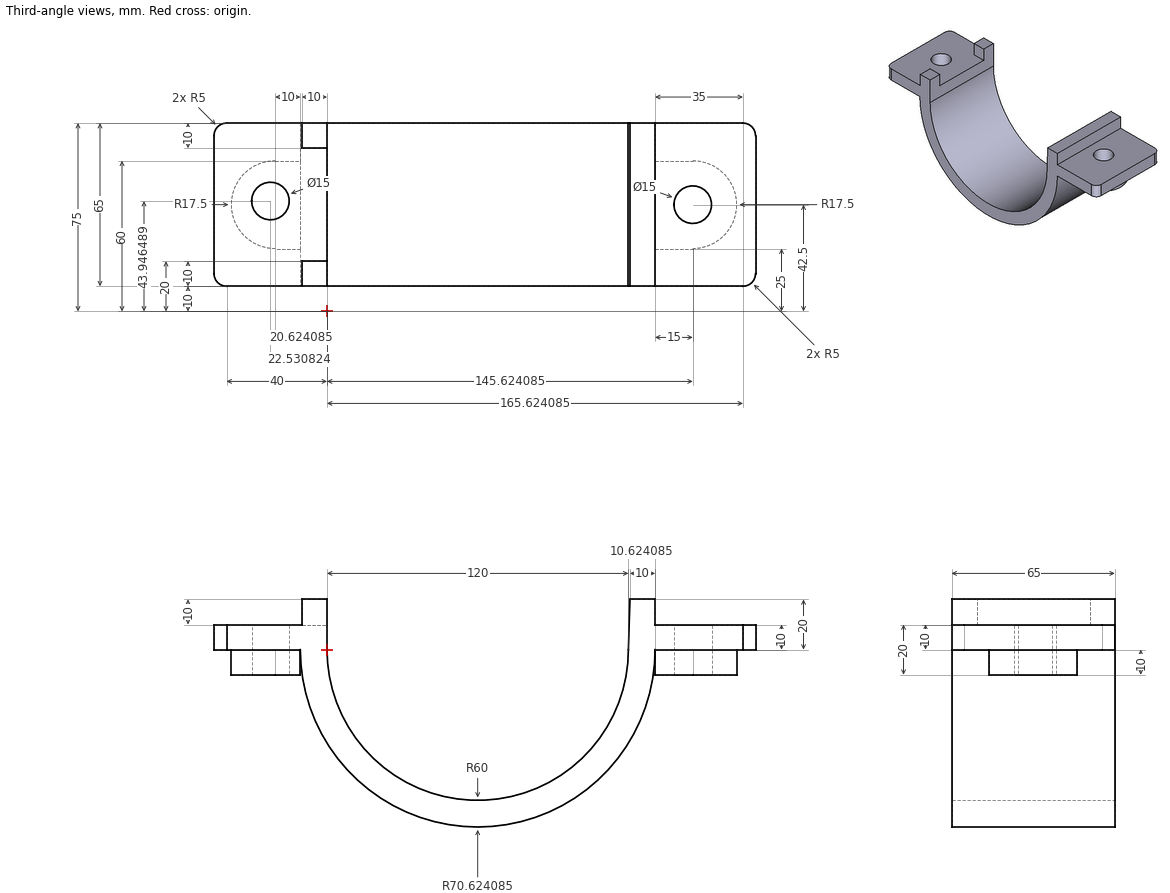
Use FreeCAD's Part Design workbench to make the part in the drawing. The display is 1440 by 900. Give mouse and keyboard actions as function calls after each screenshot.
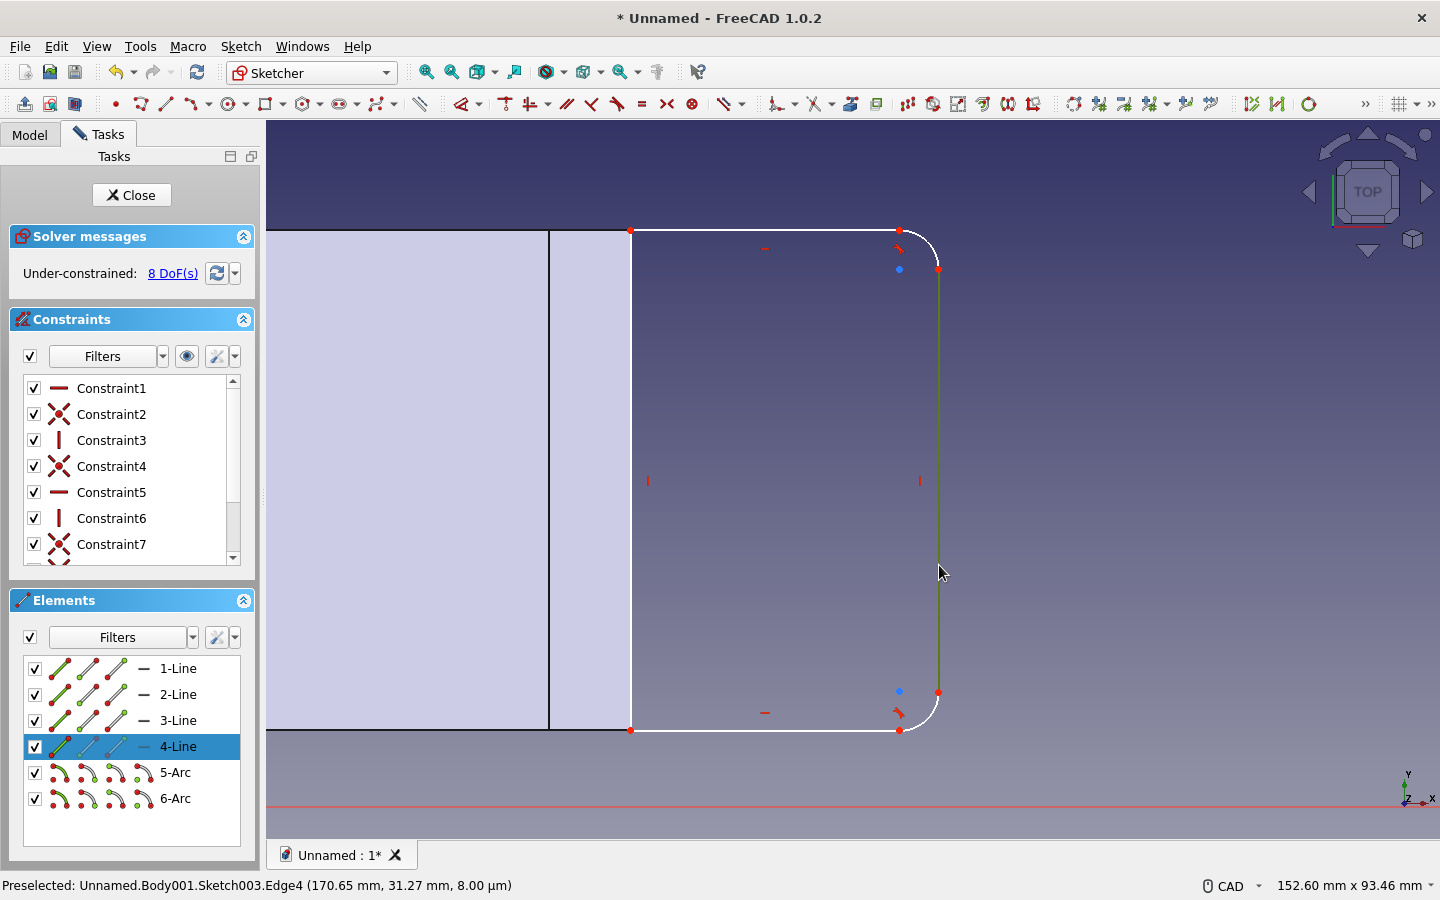
click(917, 727)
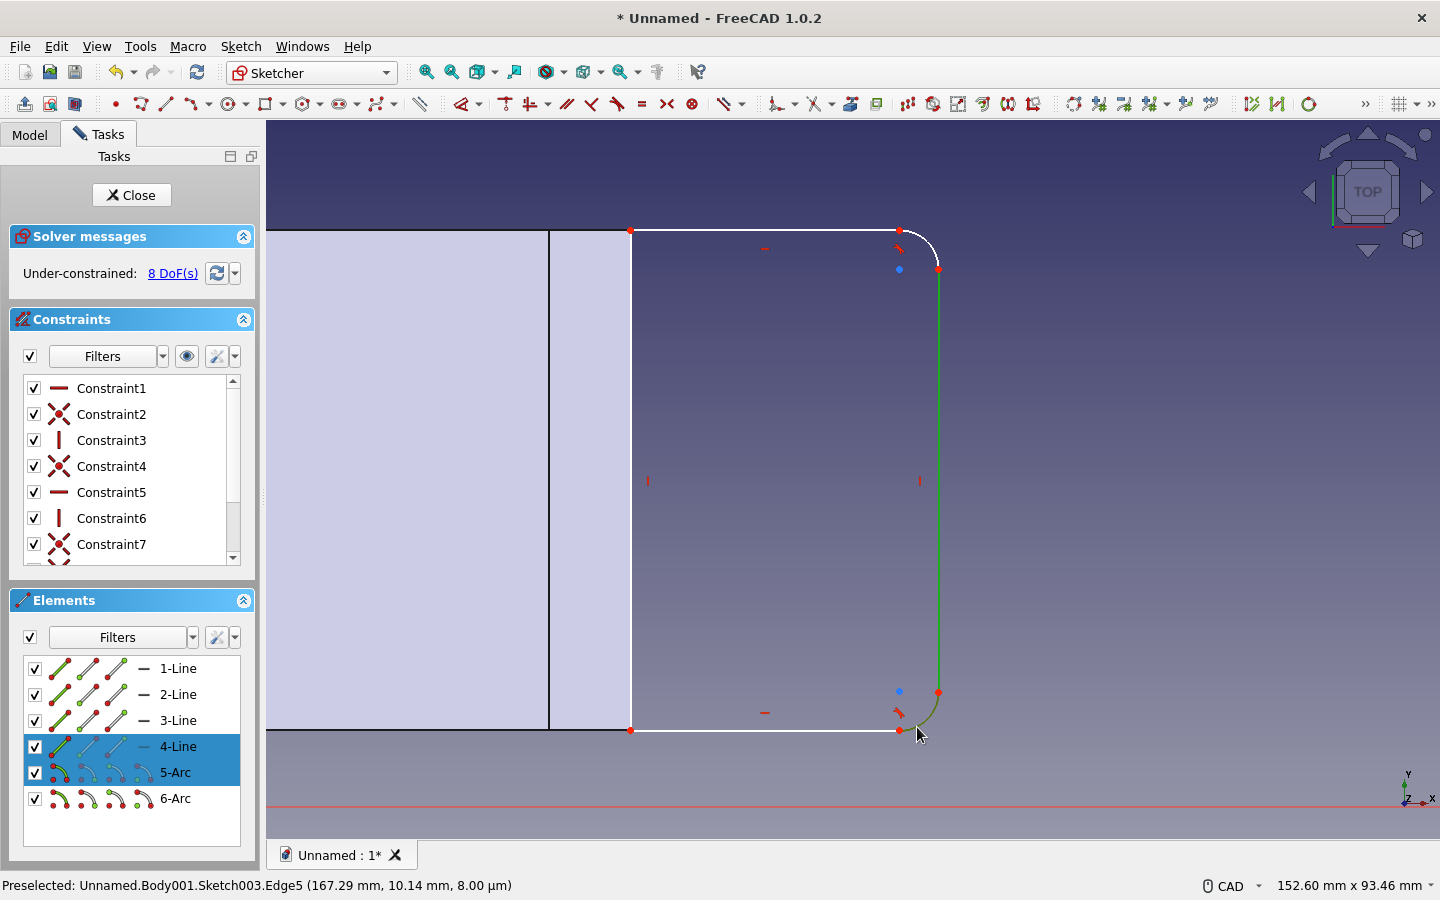
click(617, 104)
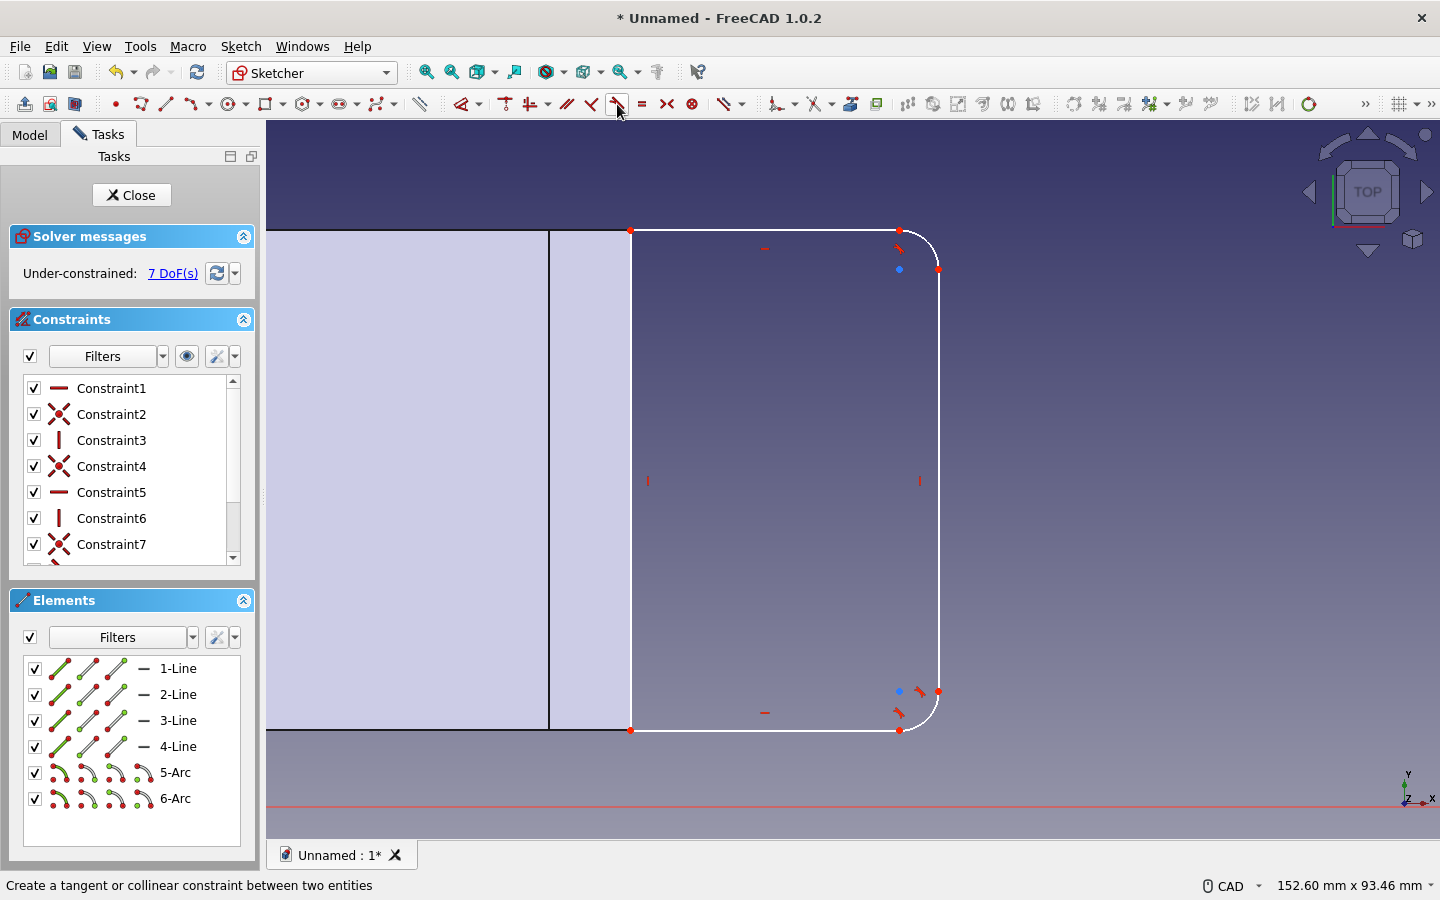
click(939, 565)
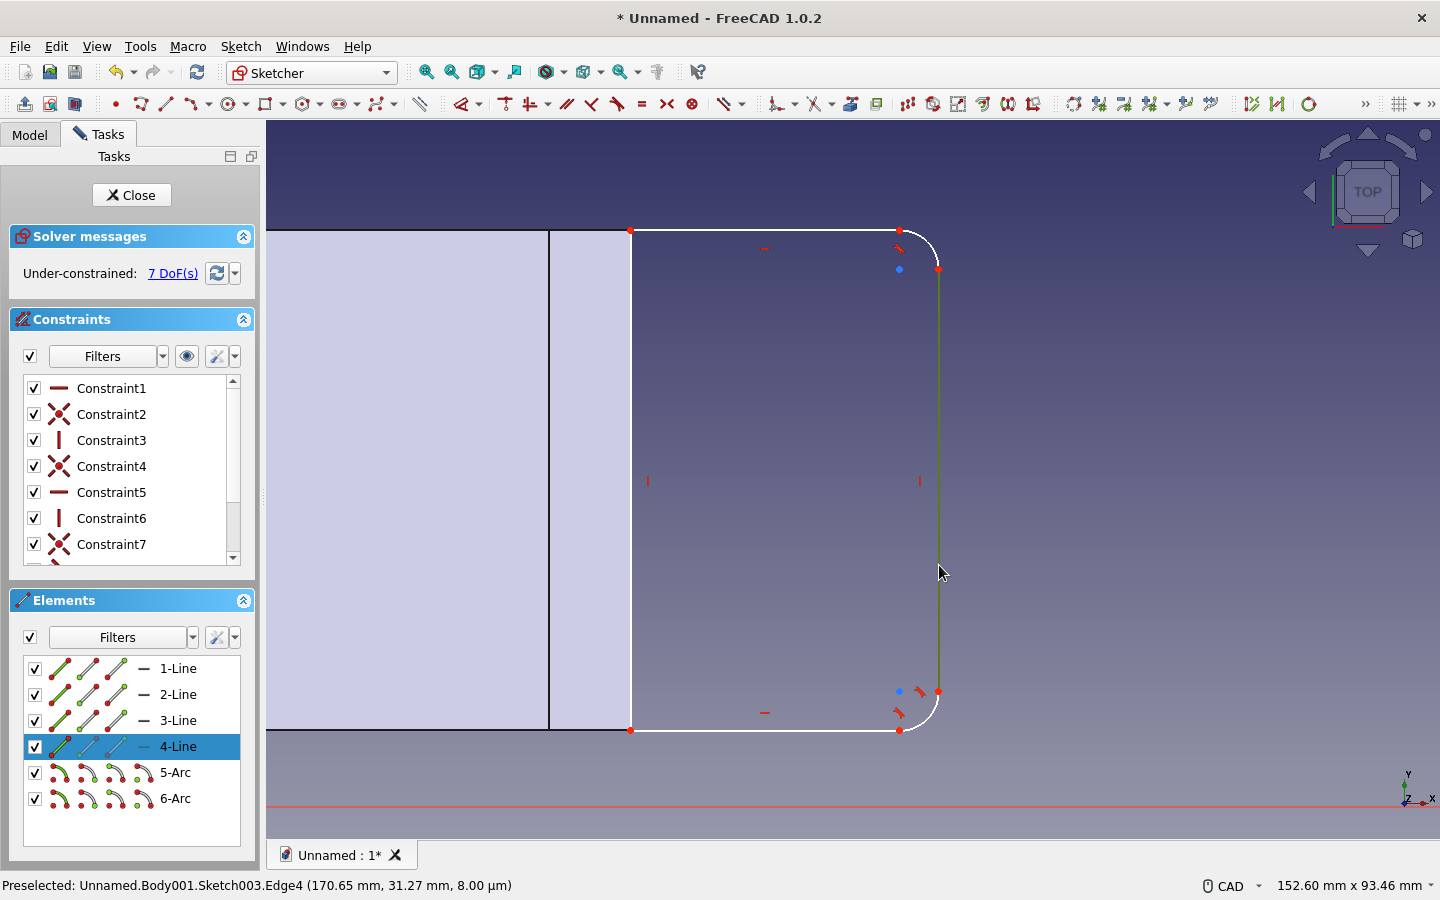
click(934, 252)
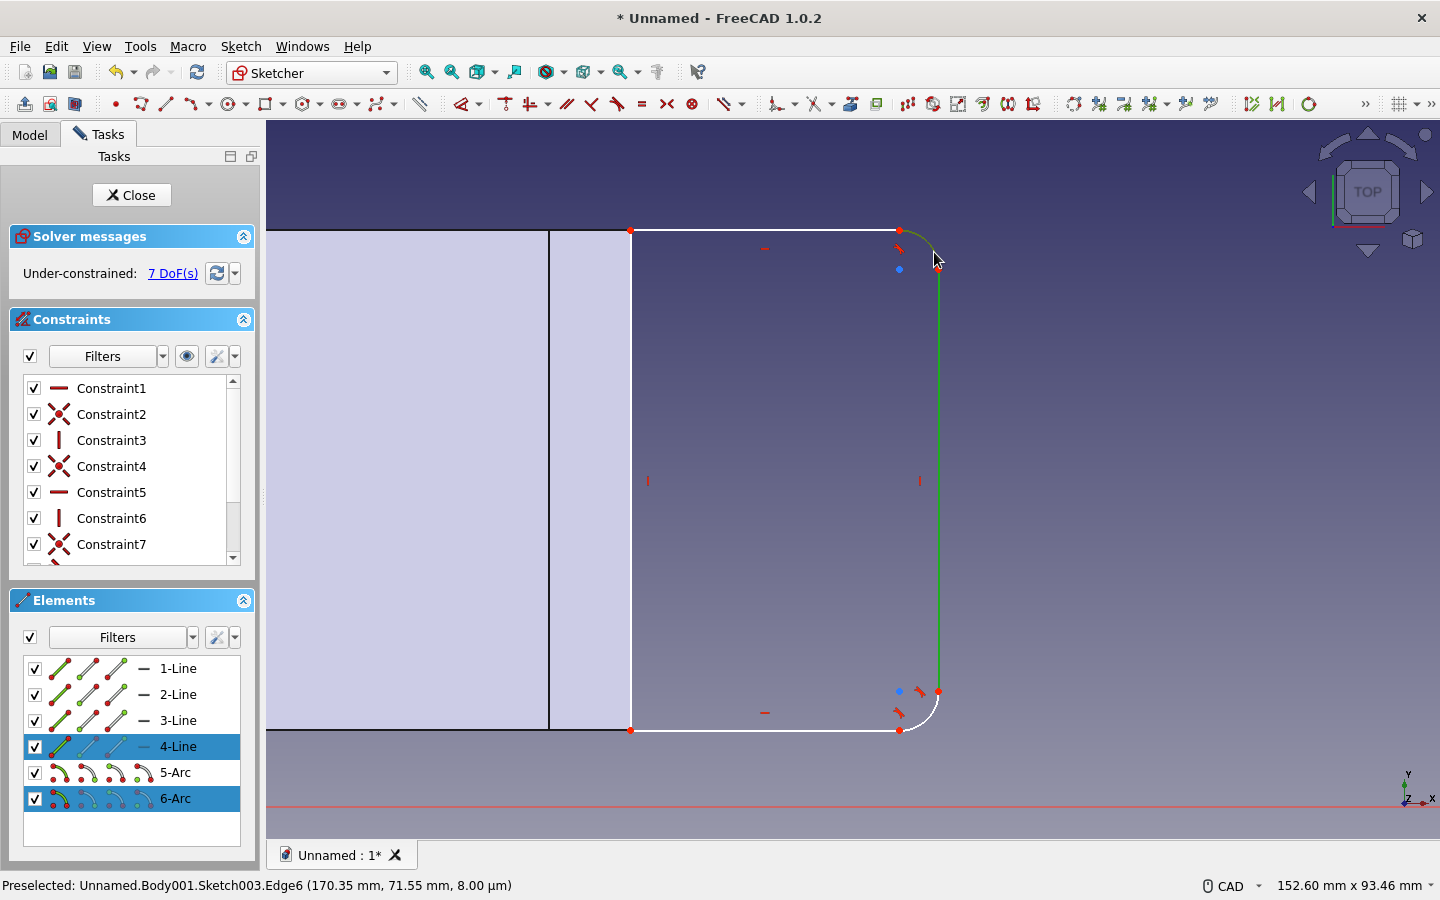
key(t)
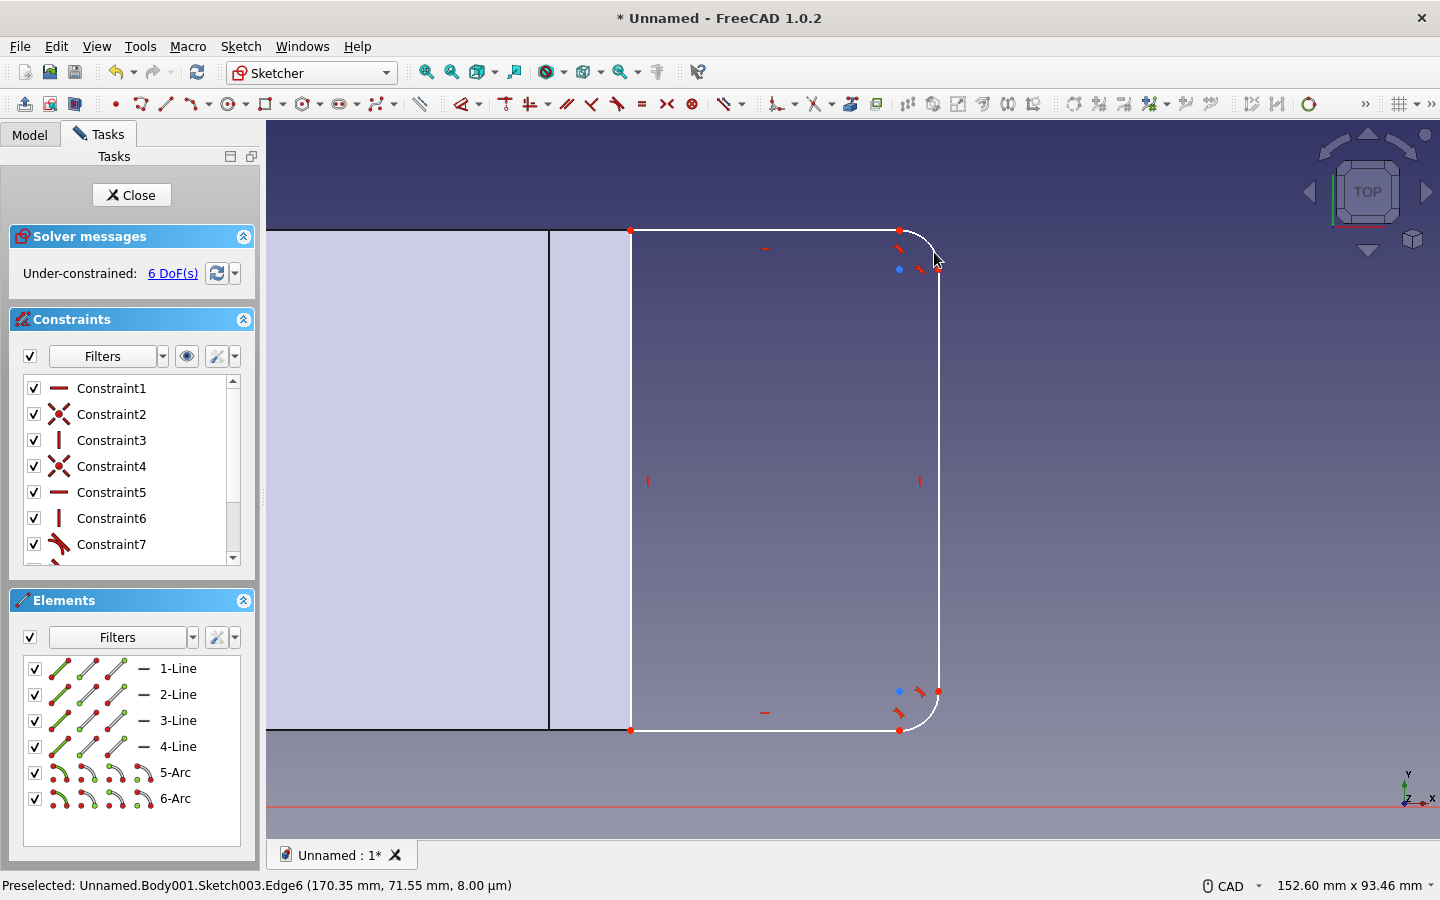
click(917, 727)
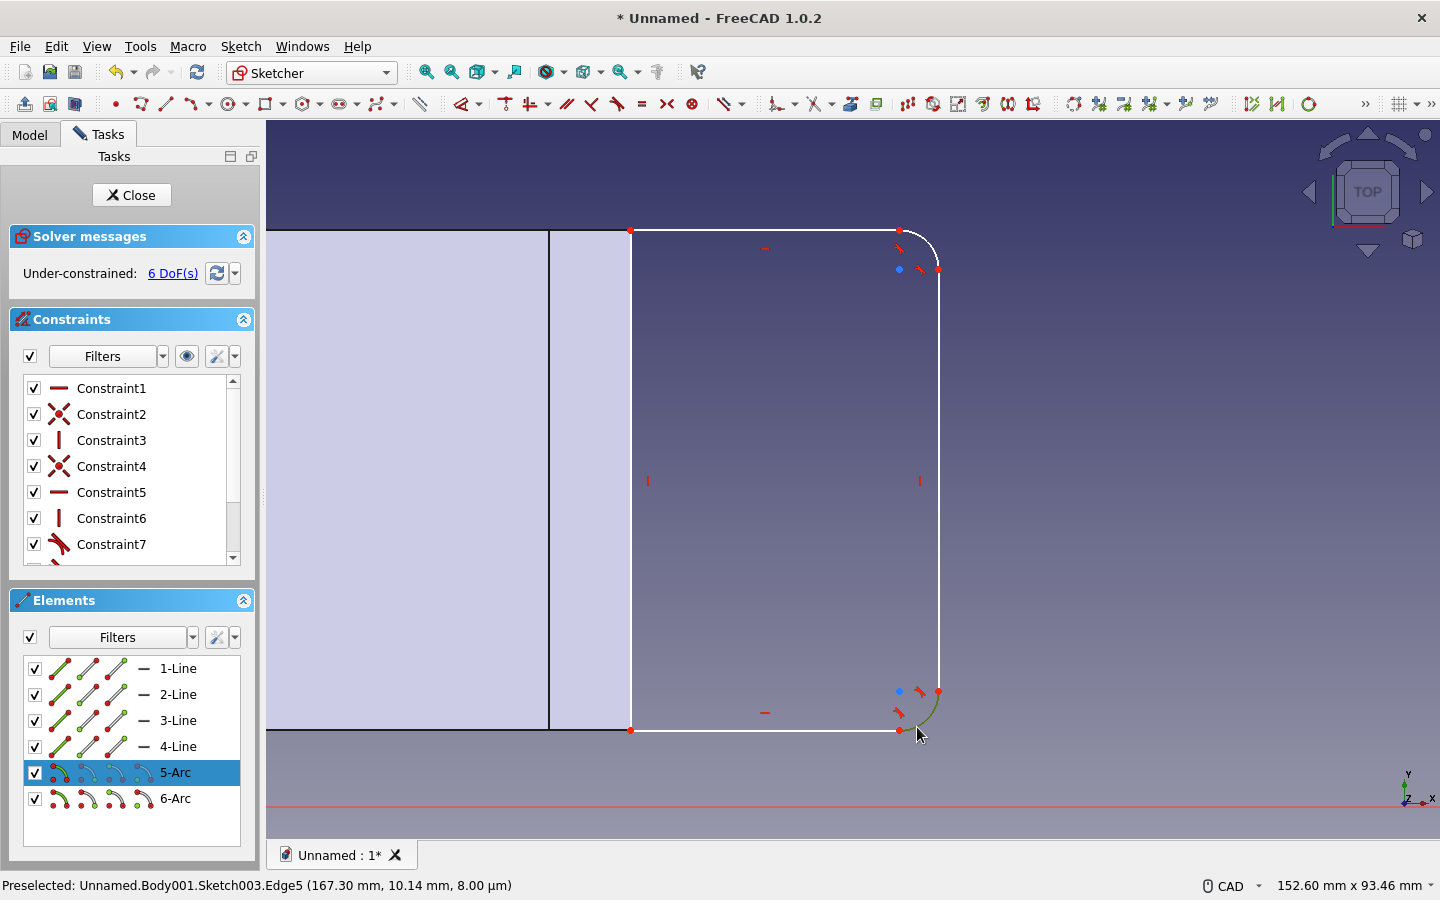
click(934, 252)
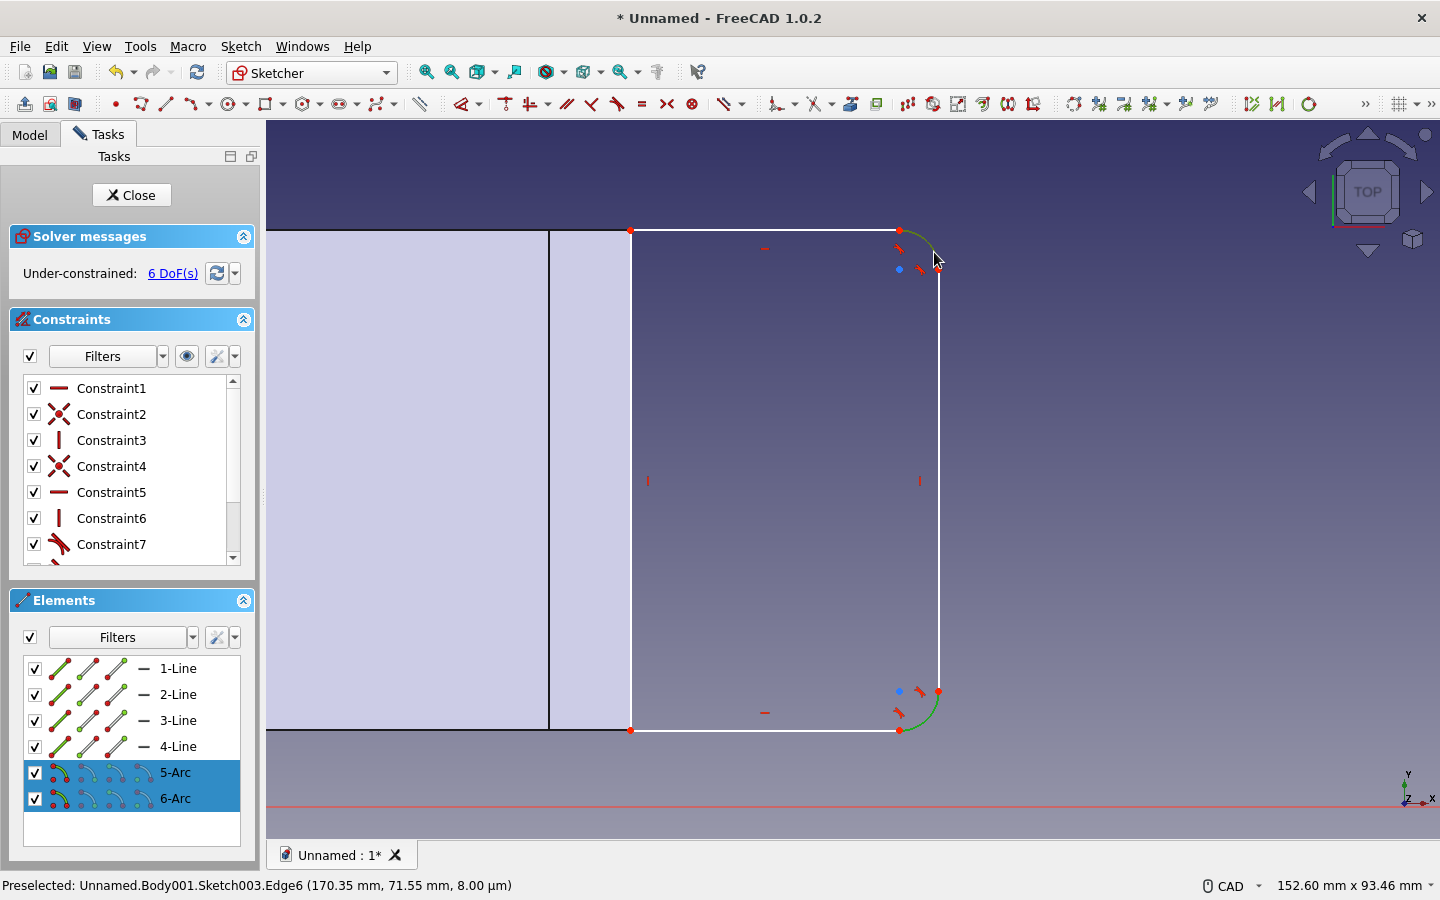
key(e)